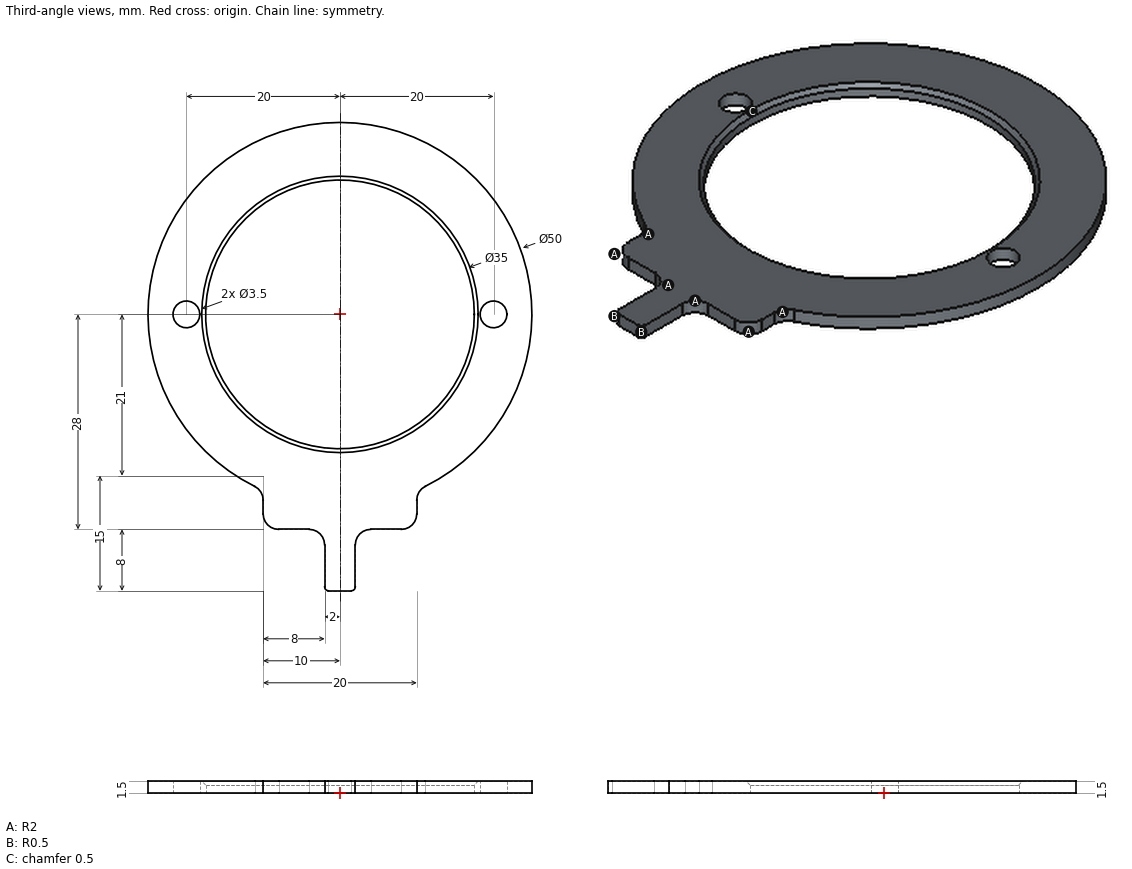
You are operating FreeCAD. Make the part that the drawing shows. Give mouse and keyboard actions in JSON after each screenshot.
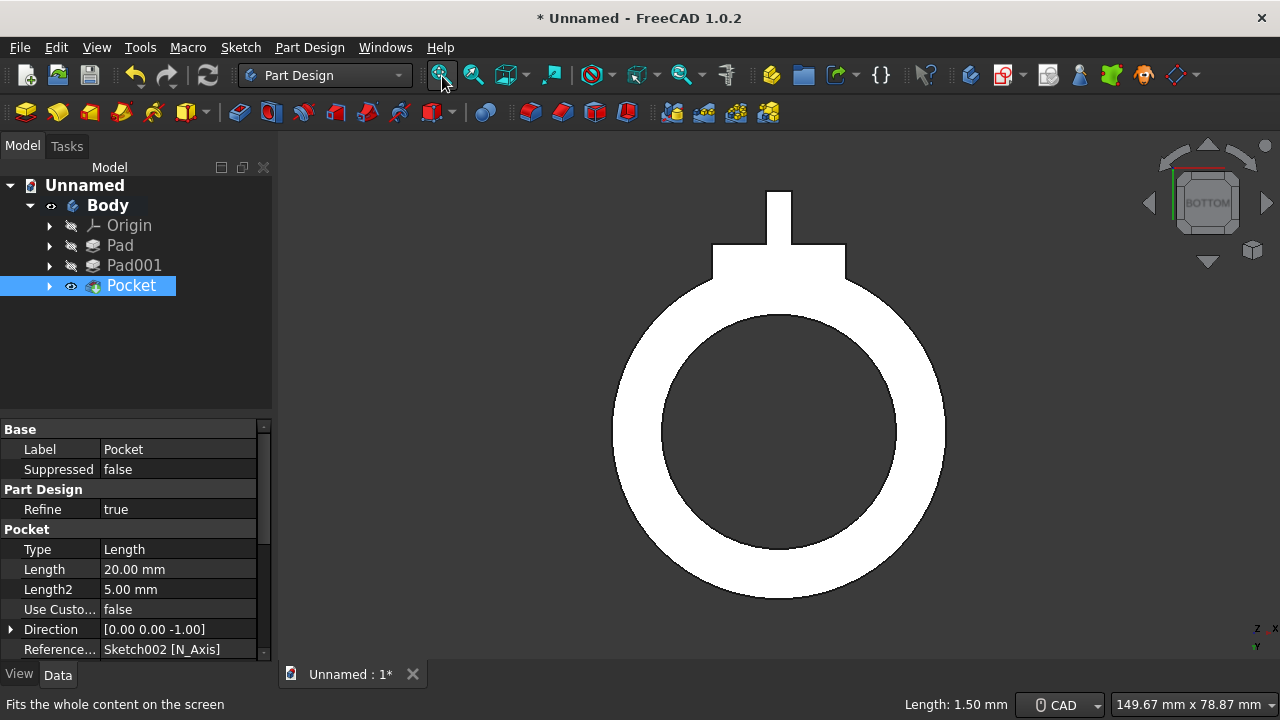
{"action": "scroll", "coordinate": [846, 277], "scroll_direction": "up", "scroll_amount": 7}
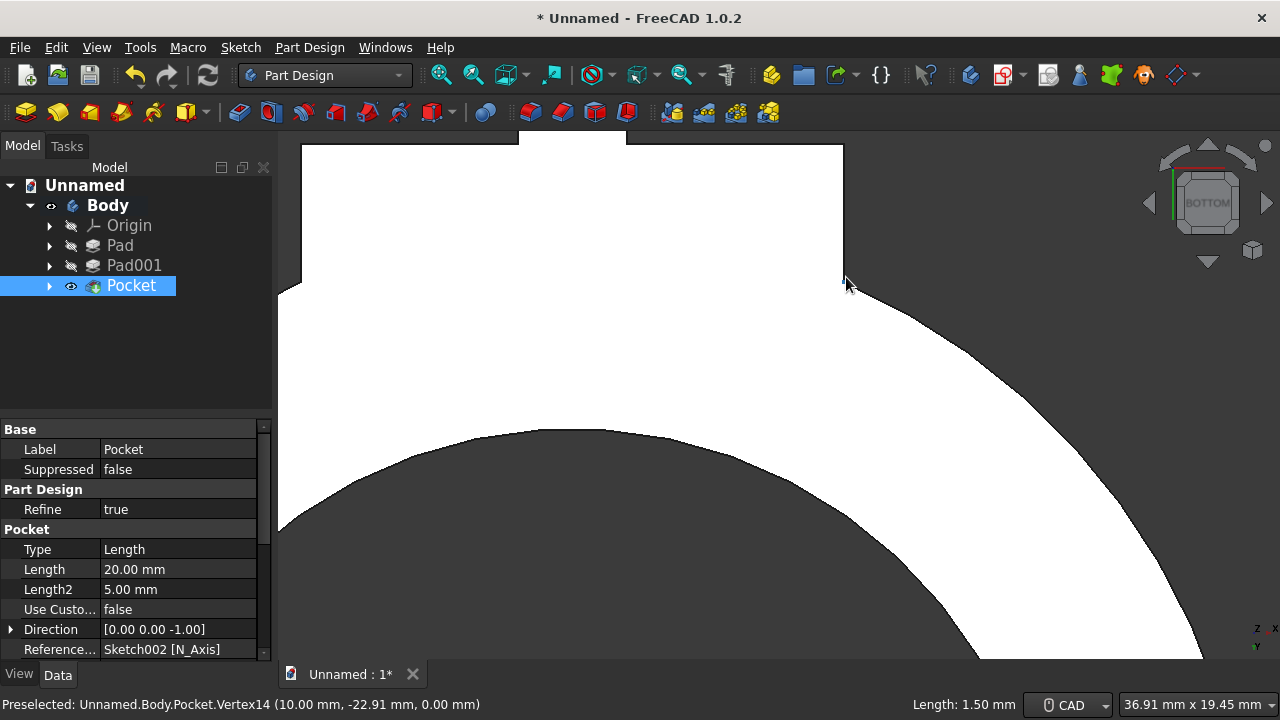
{"action": "left_click", "coordinate": [442, 76]}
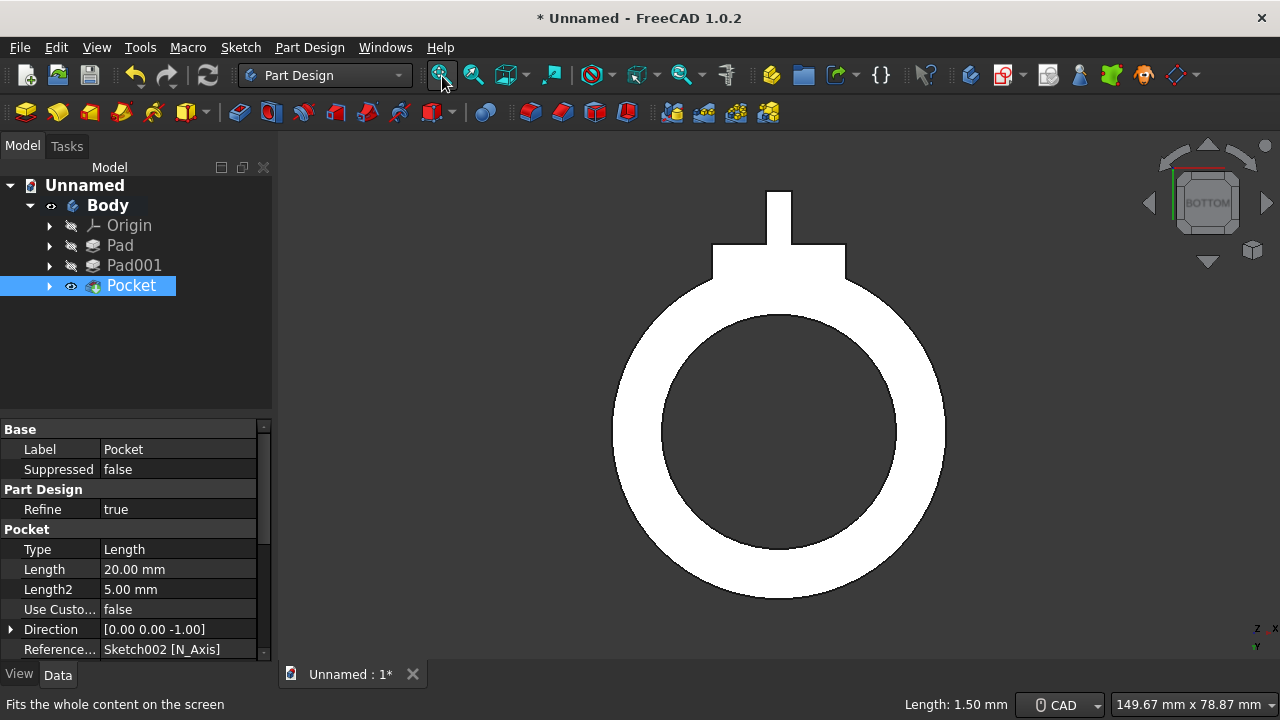
{"action": "key", "text": "4"}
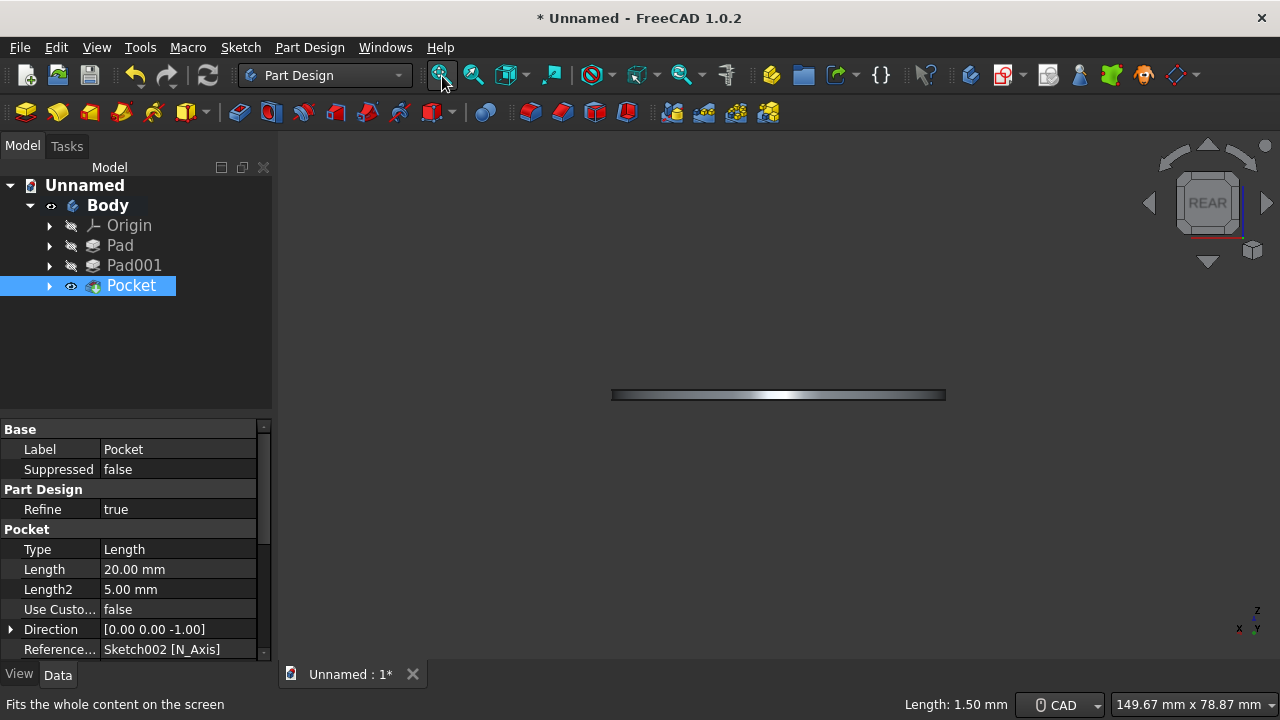
{"action": "left_click", "coordinate": [442, 76]}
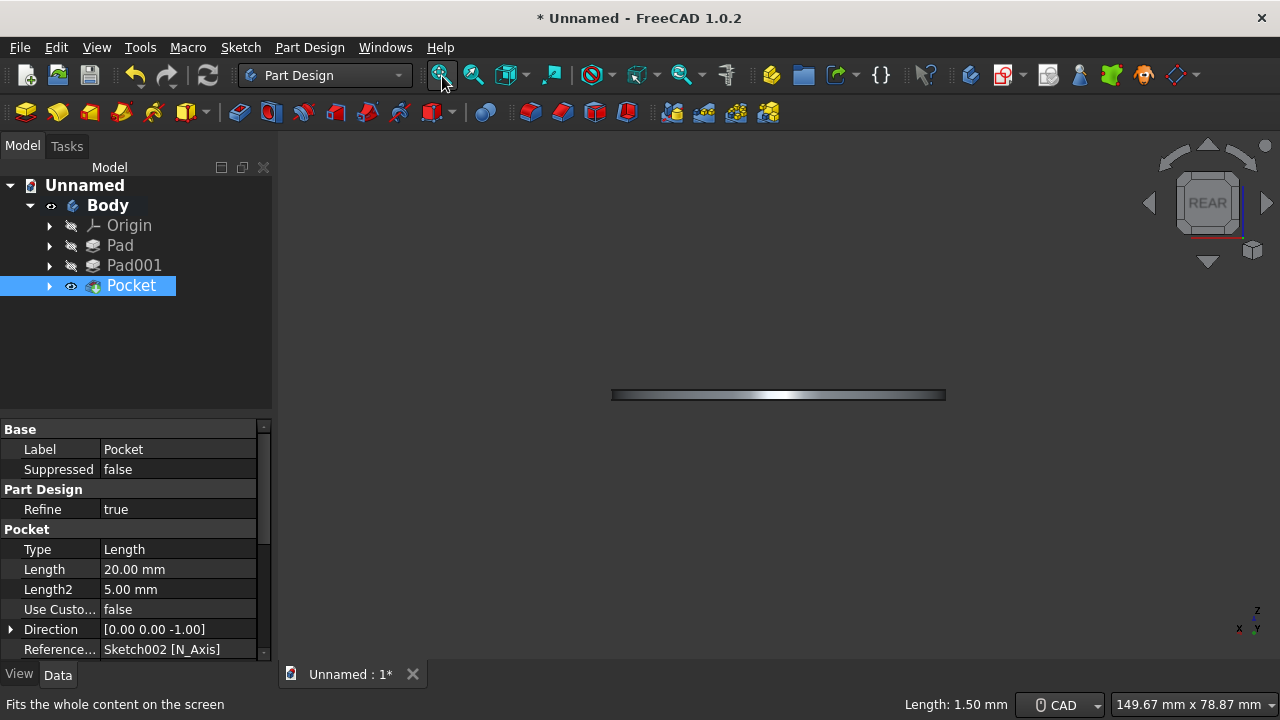
{"action": "scroll", "coordinate": [712, 394], "scroll_direction": "up", "scroll_amount": 7}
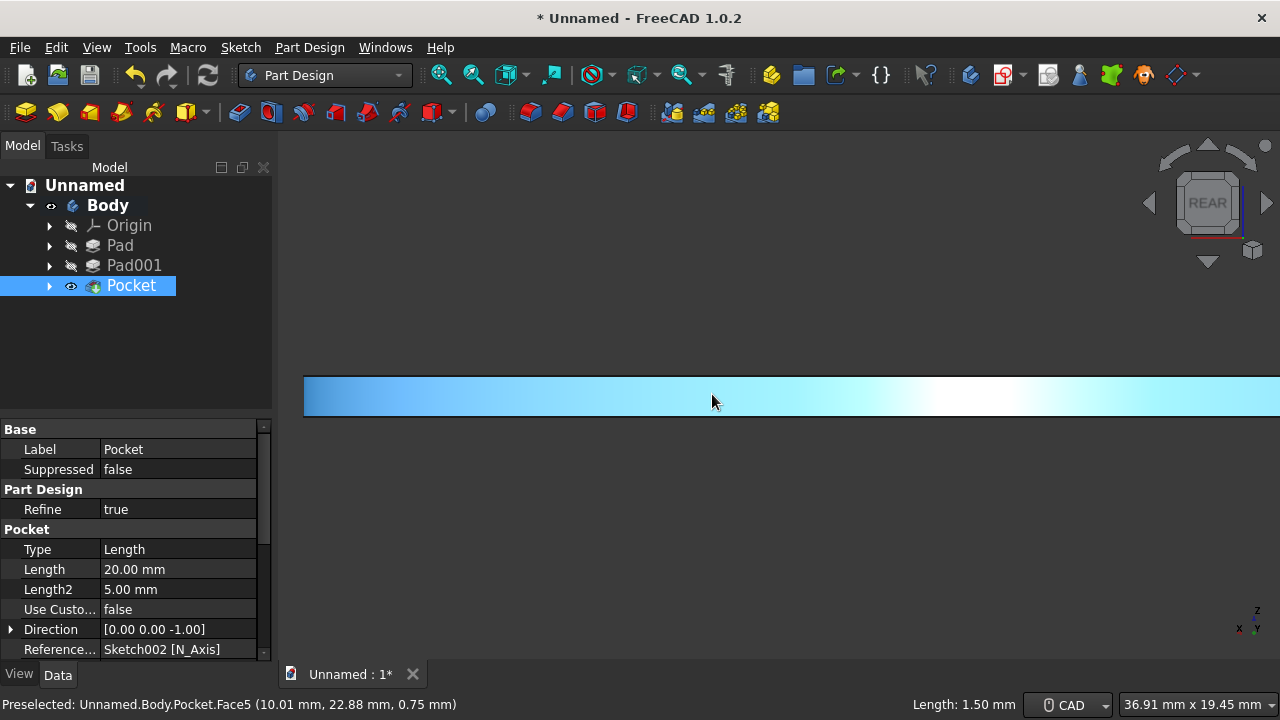
{"action": "left_click", "coordinate": [442, 76]}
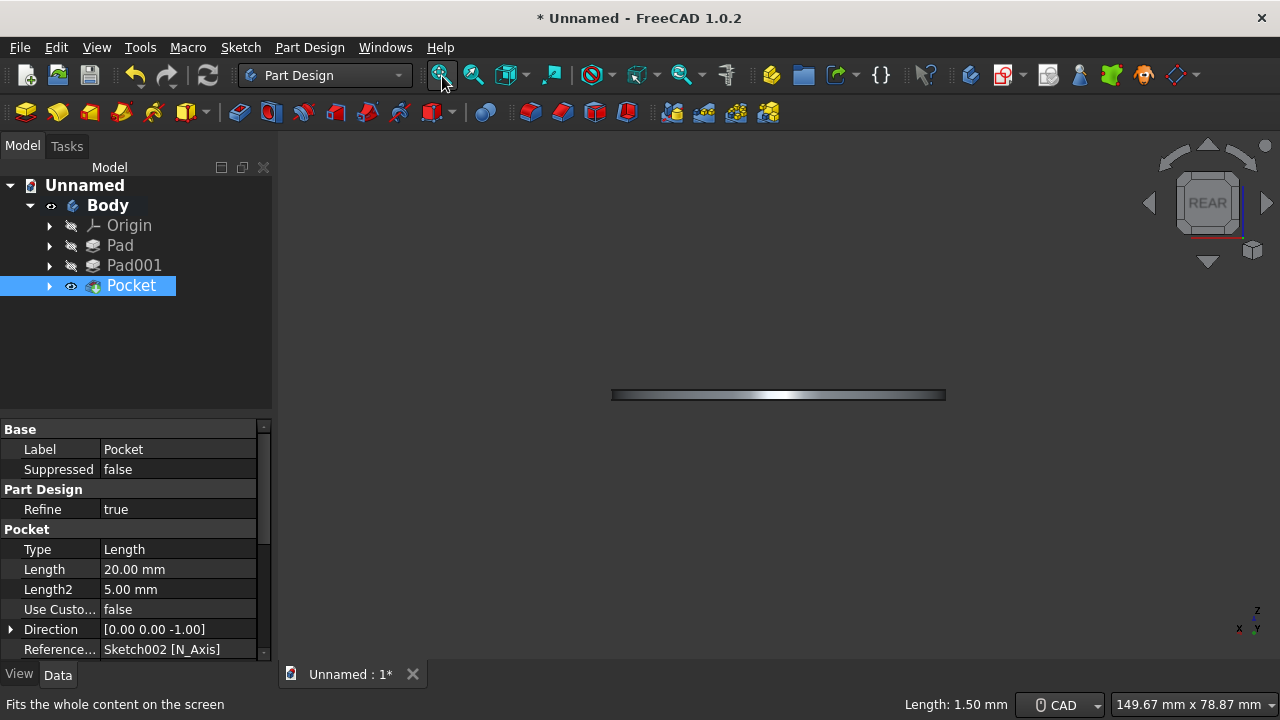
{"action": "key", "text": "6"}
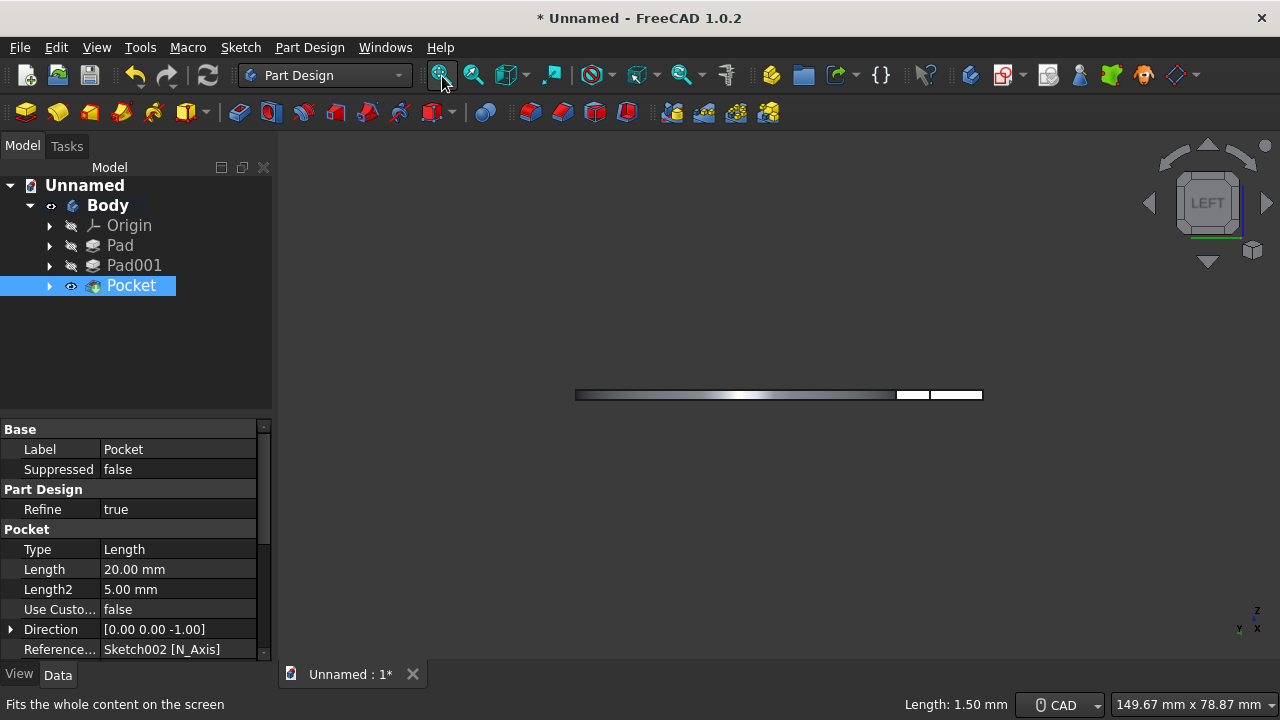
{"action": "left_click", "coordinate": [442, 76]}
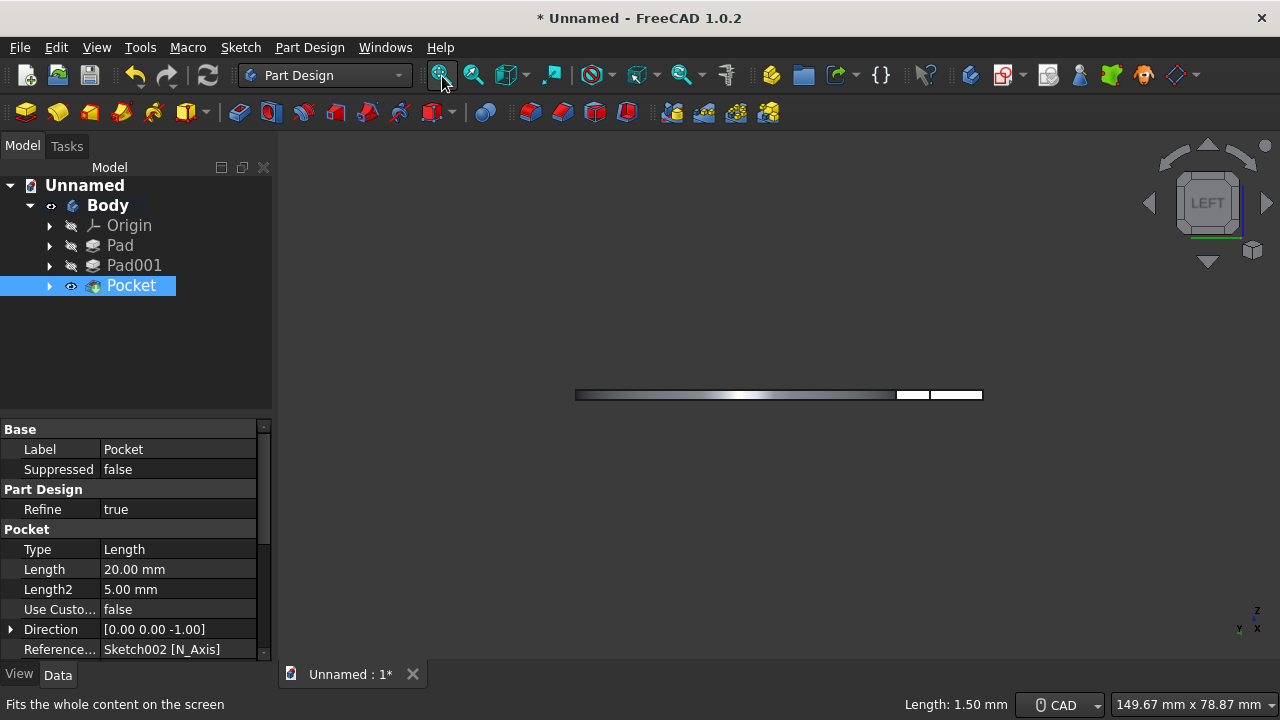
{"action": "scroll", "coordinate": [896, 394], "scroll_direction": "up", "scroll_amount": 7}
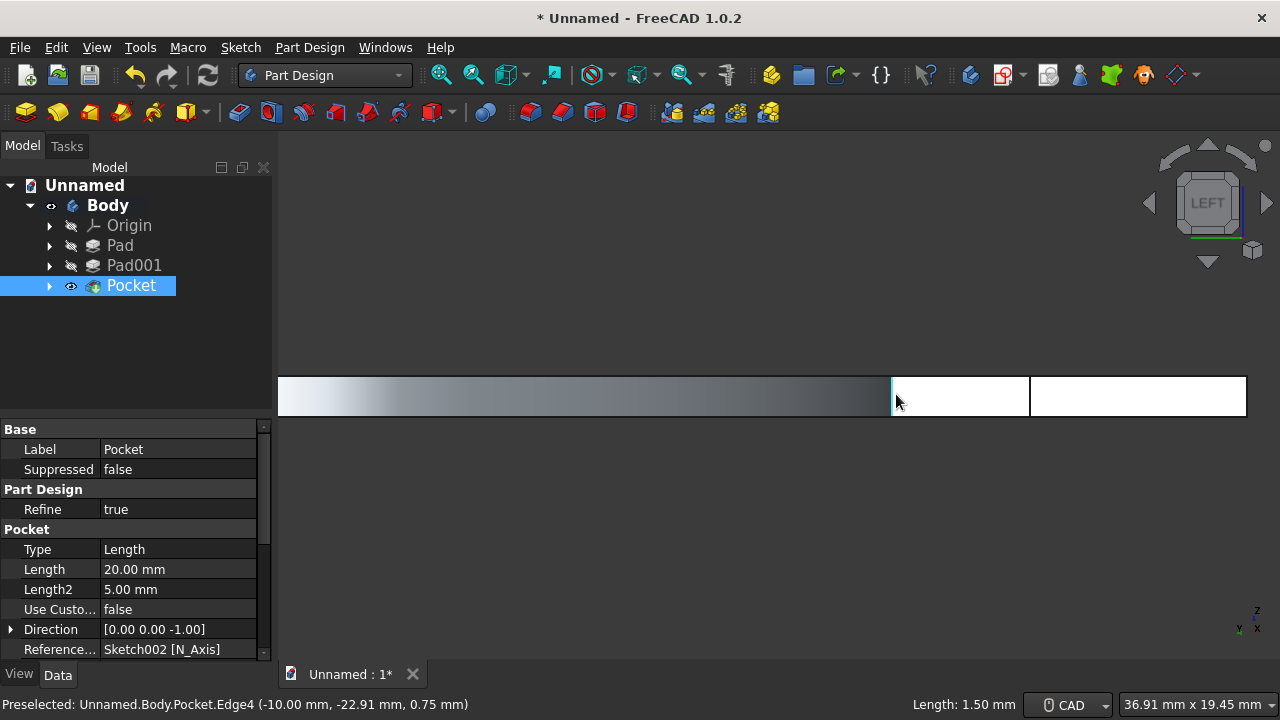
{"action": "left_click", "coordinate": [1030, 396], "text": "ctrl"}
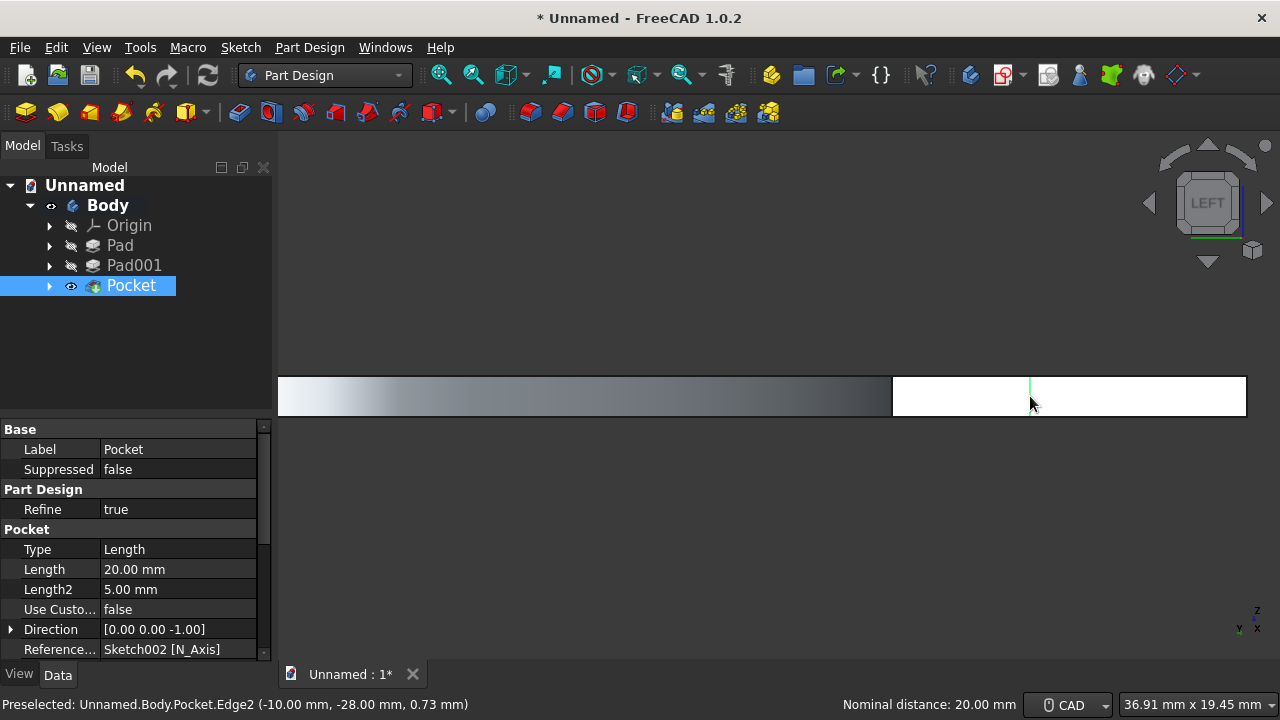
{"action": "left_click", "coordinate": [442, 76]}